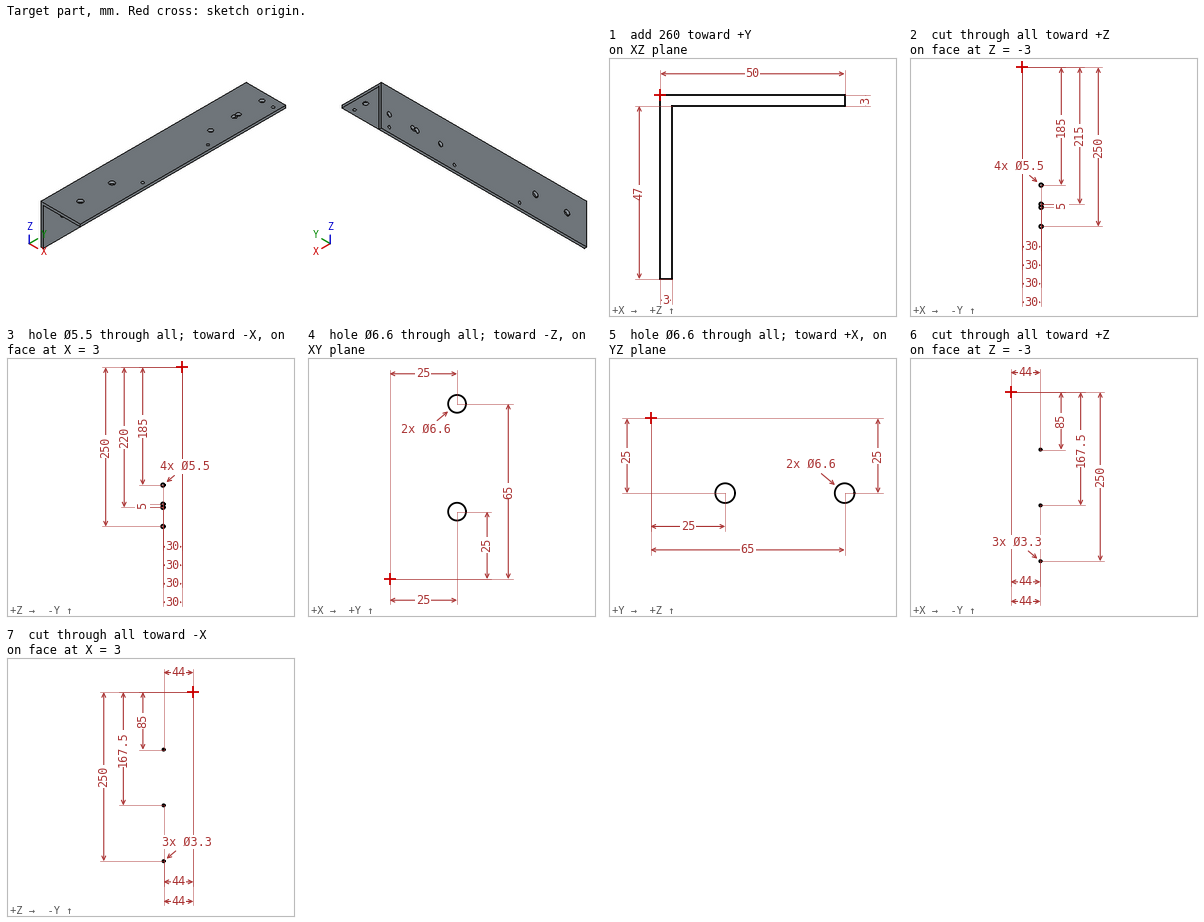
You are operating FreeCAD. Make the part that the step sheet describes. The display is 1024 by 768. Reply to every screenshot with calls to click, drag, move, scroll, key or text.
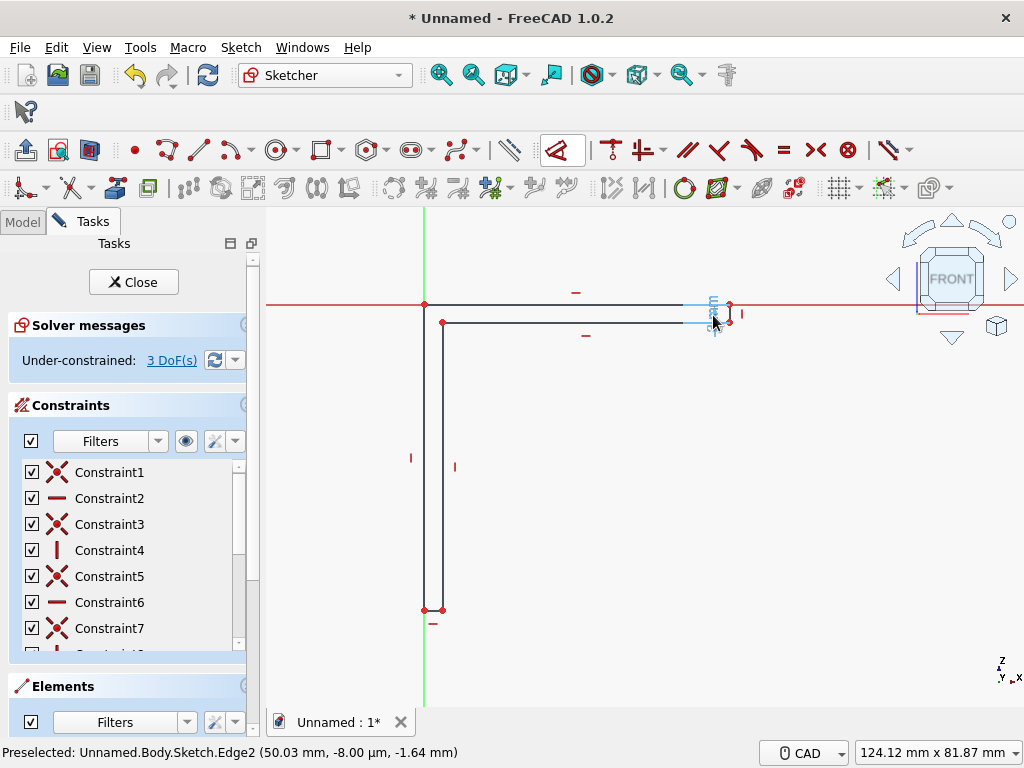
scroll(437, 611, up, 5)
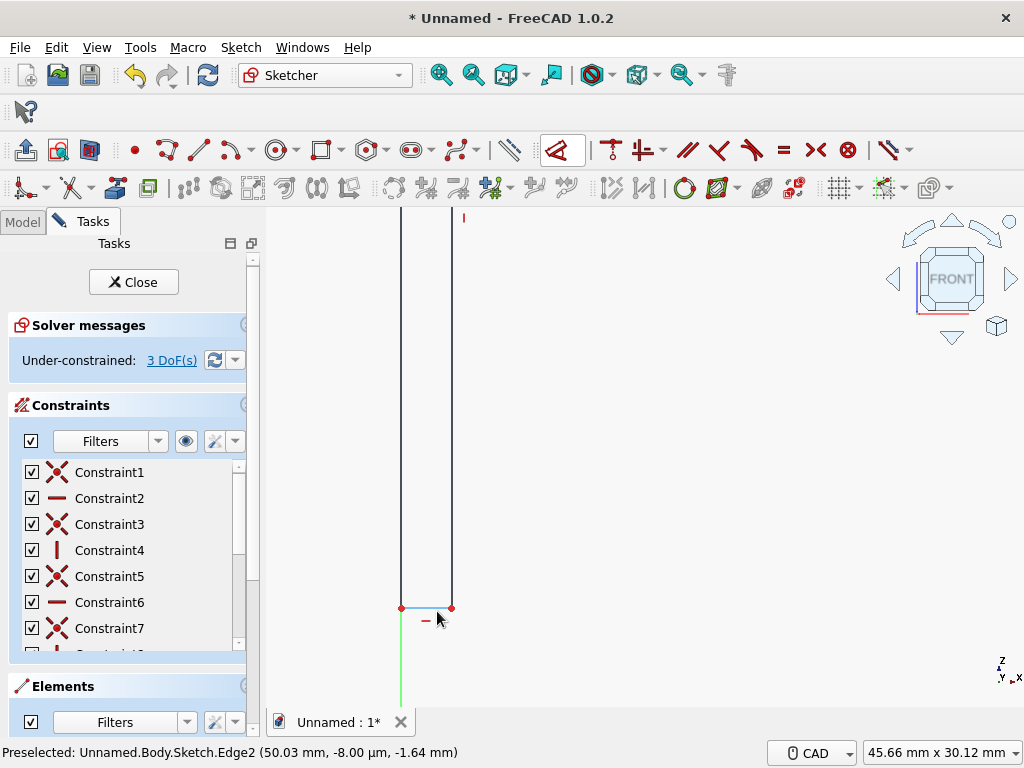
click(437, 608)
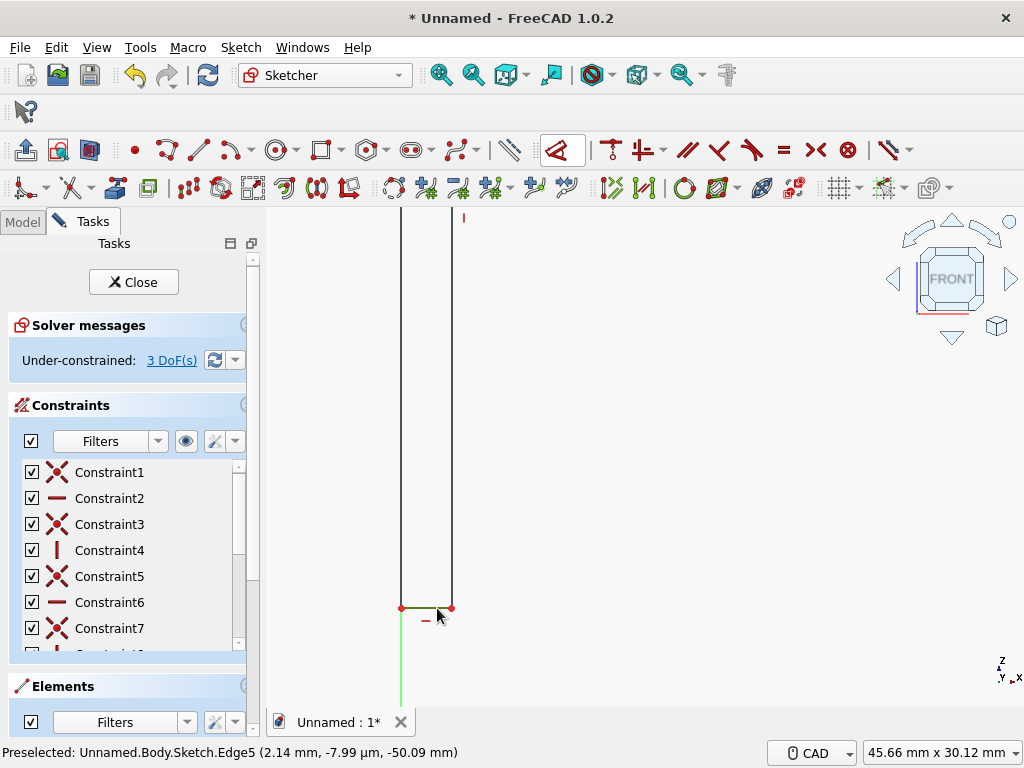
key(l)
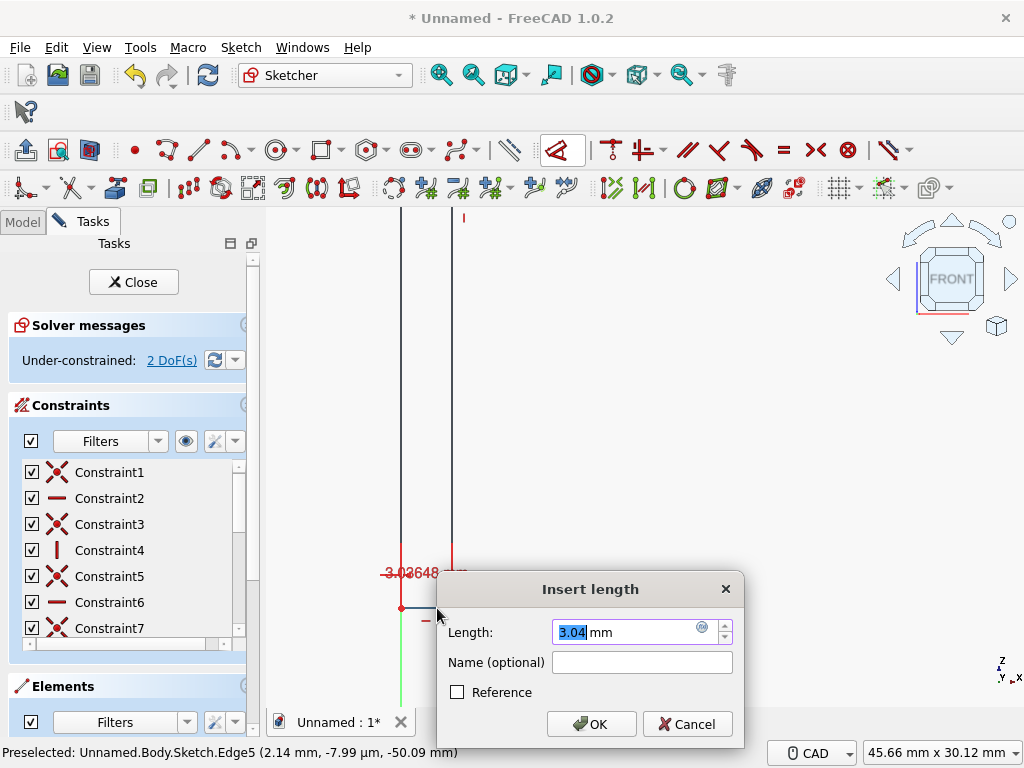
text(3)
key(Return)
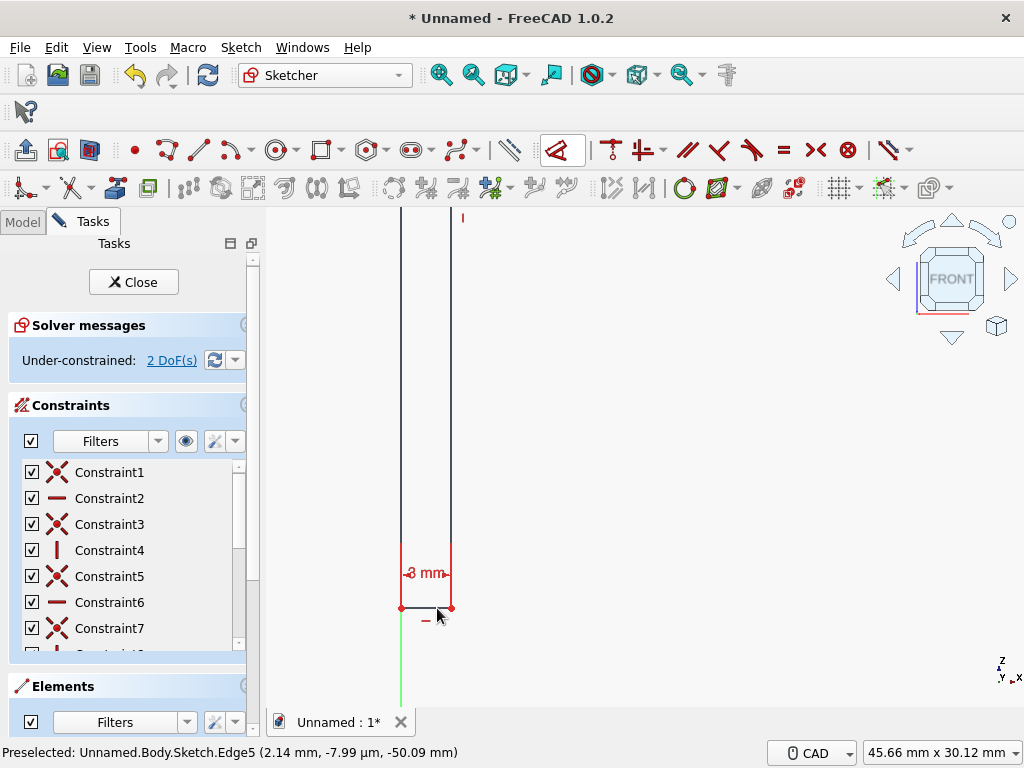
scroll(437, 611, down, 5)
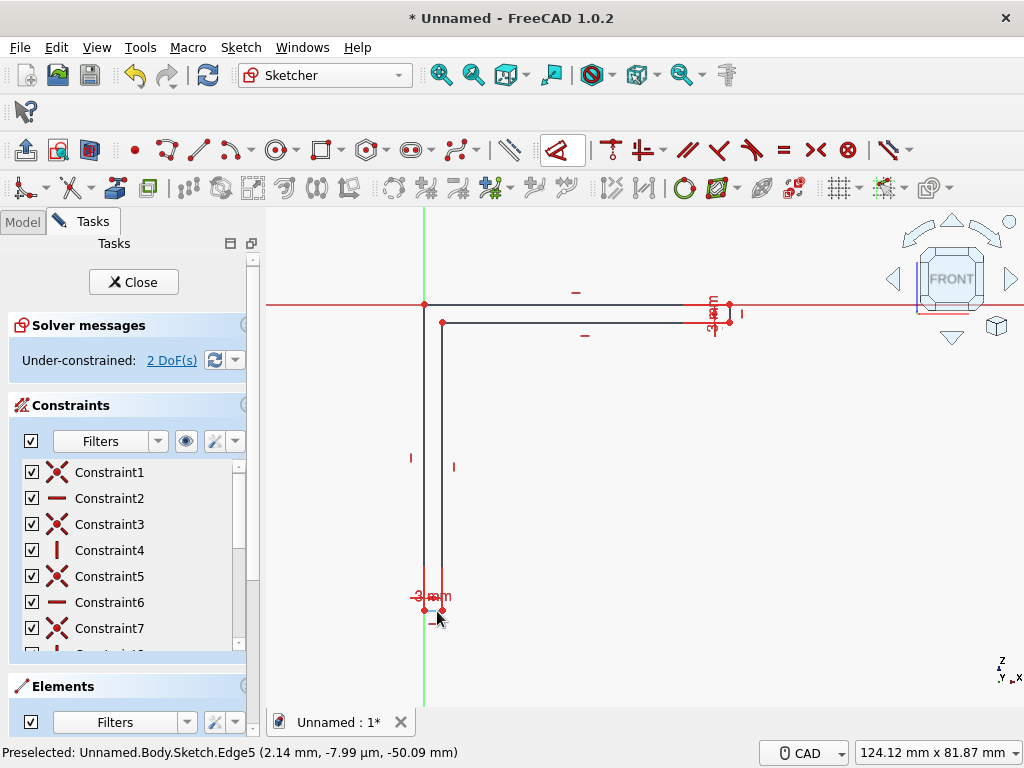
click(516, 305)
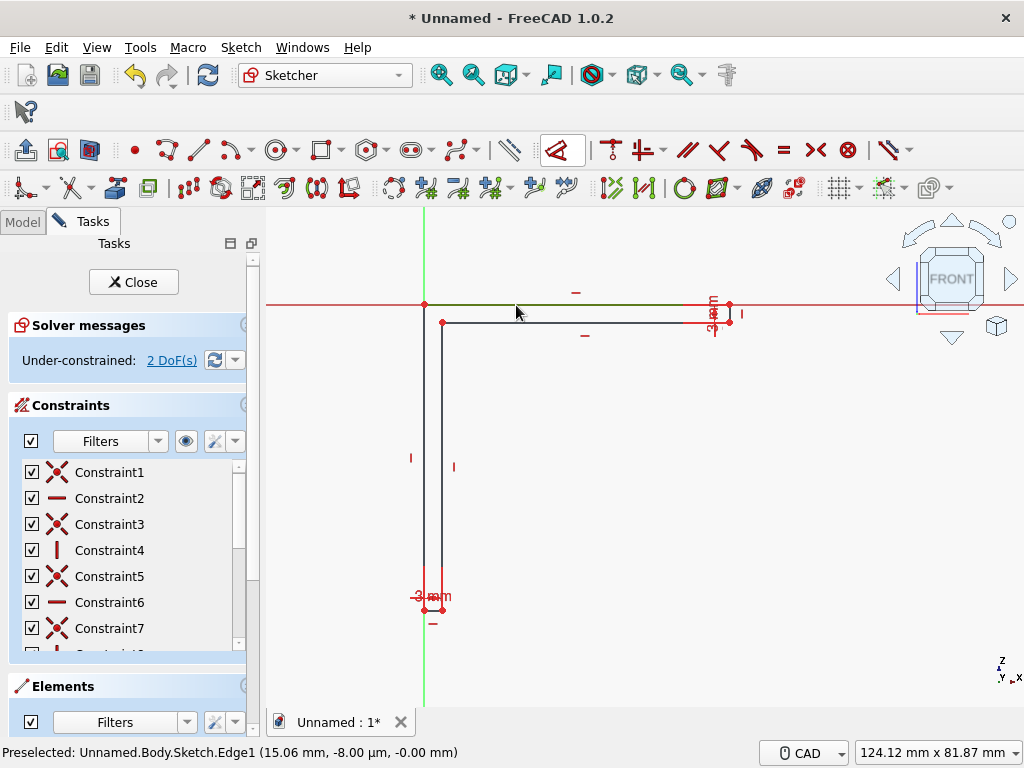
key(l)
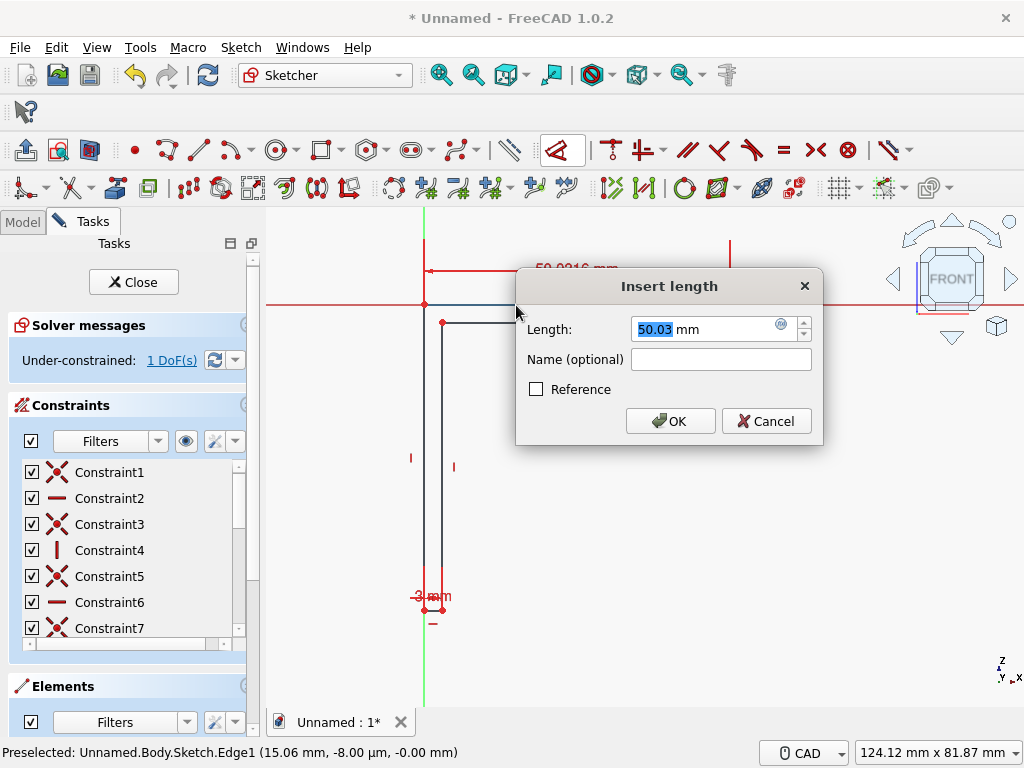
text(50)
key(Return)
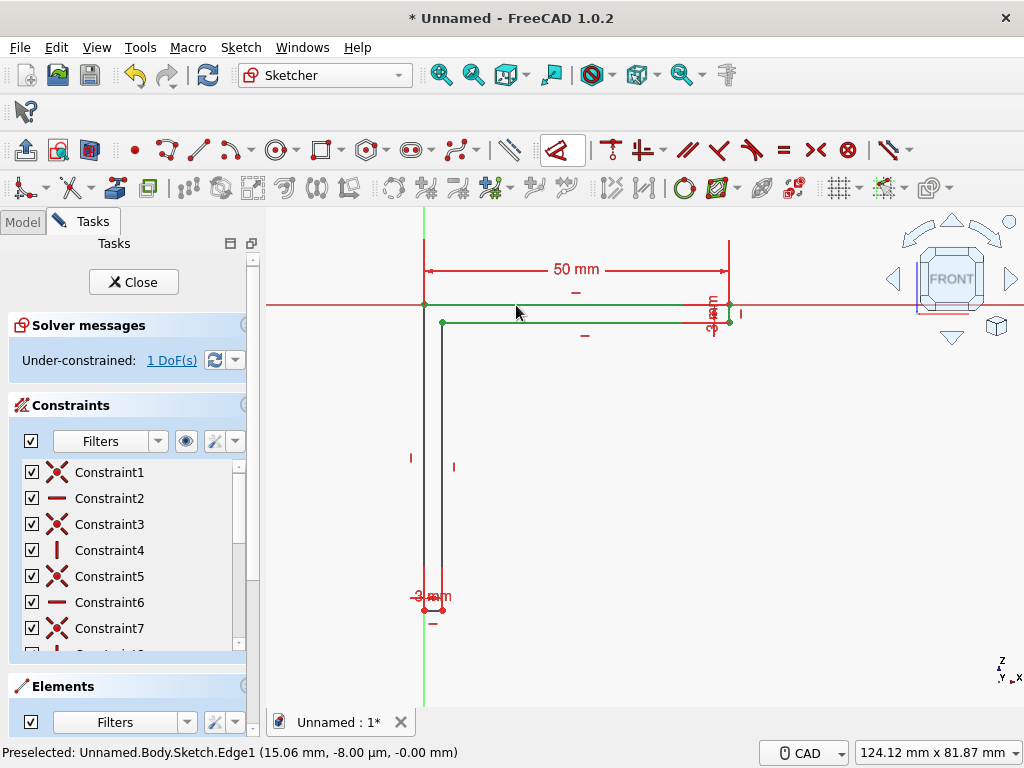
click(442, 409)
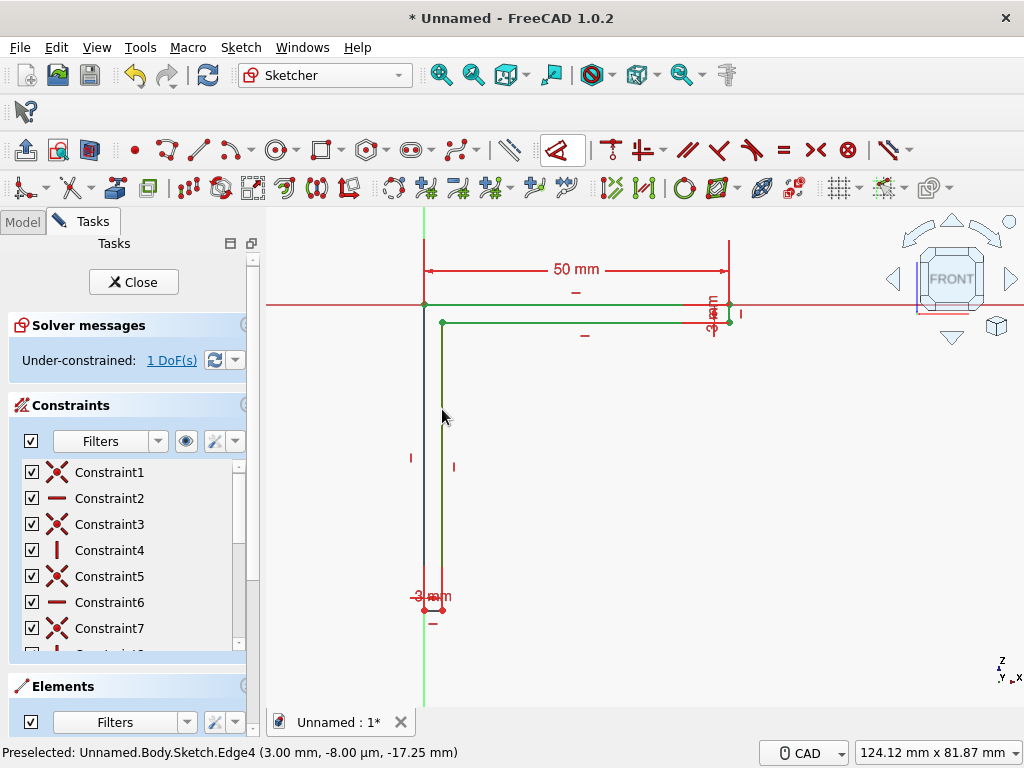
key(i)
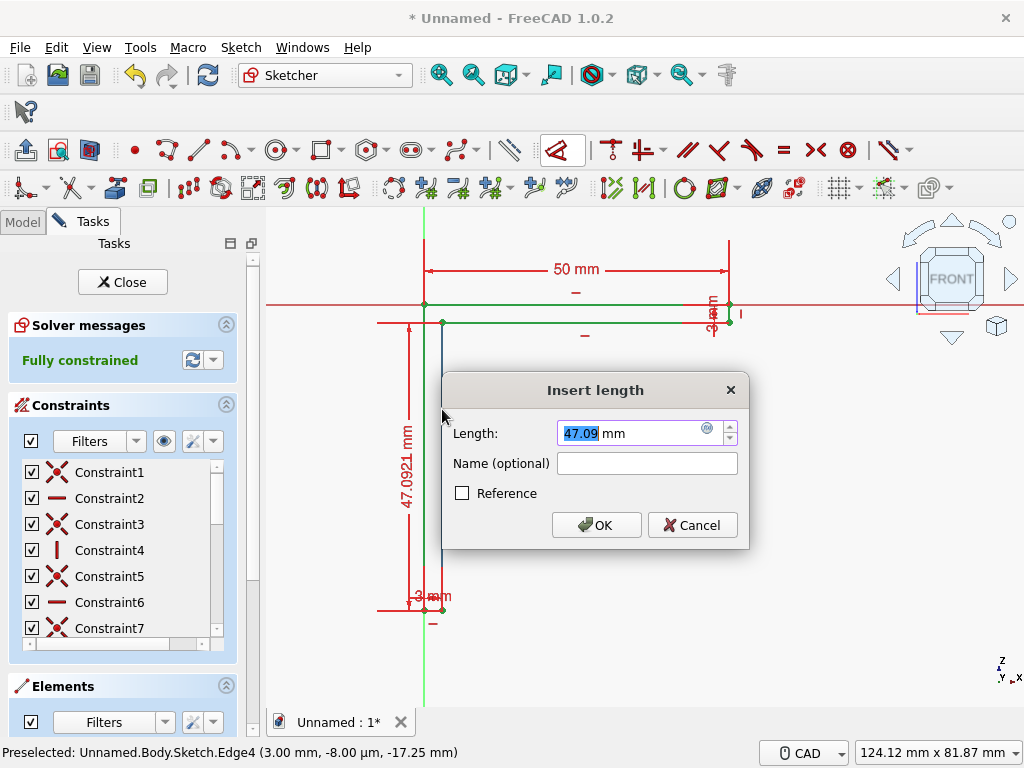
text(47)
key(Return)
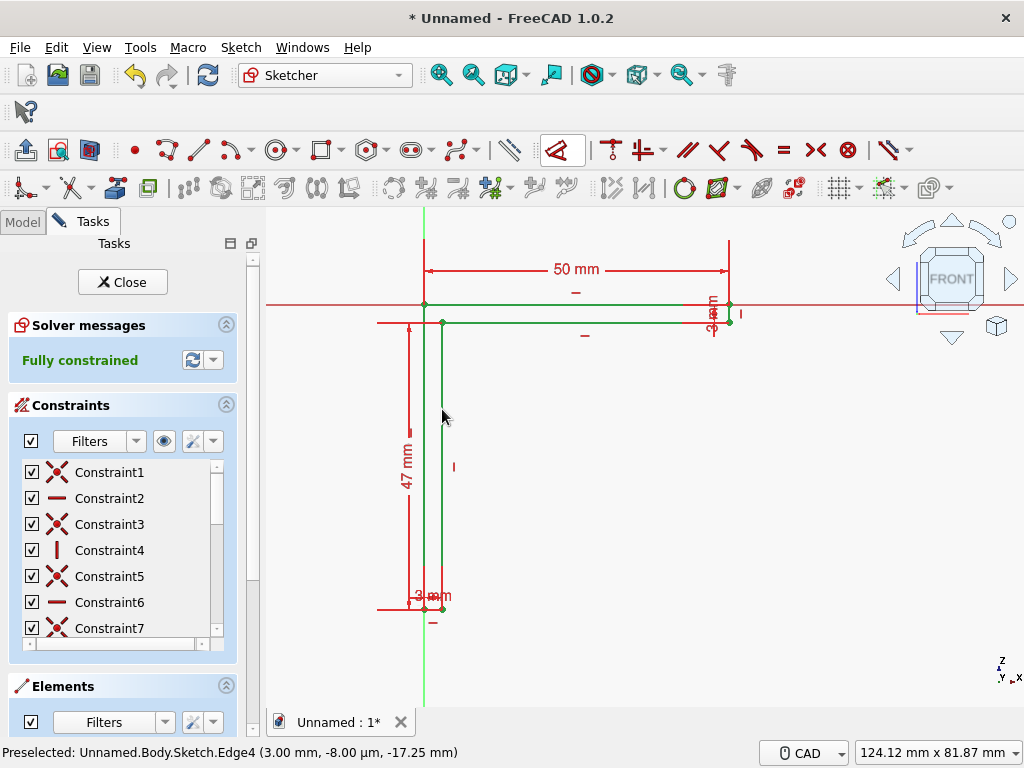
click(123, 282)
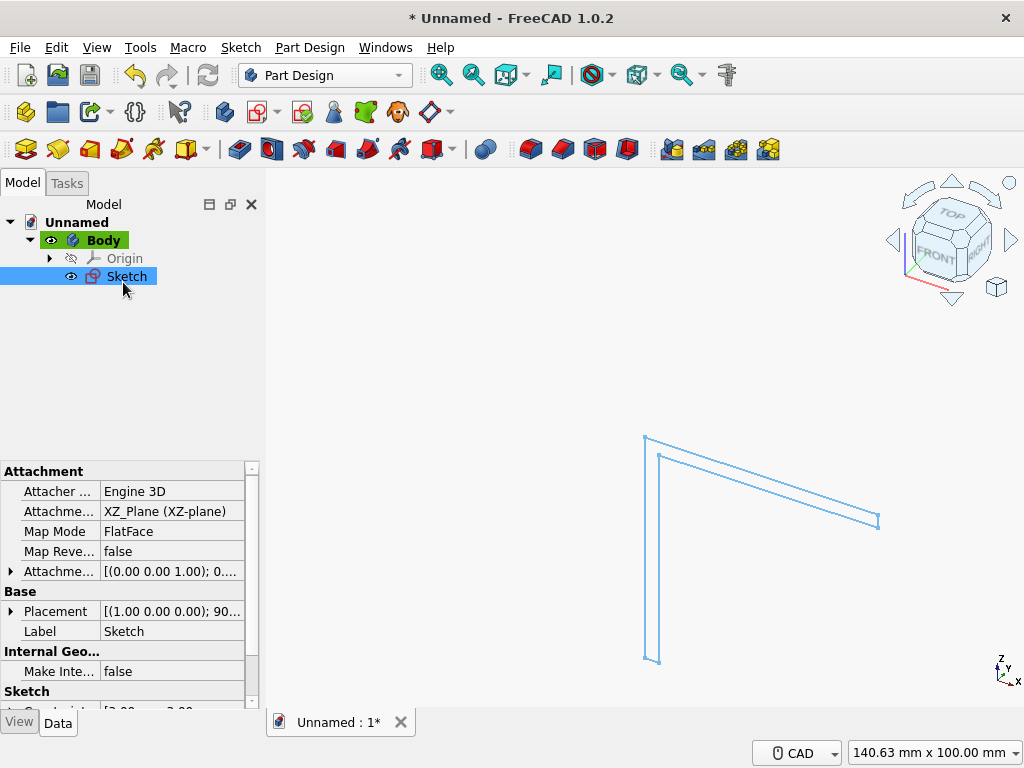
click(26, 150)